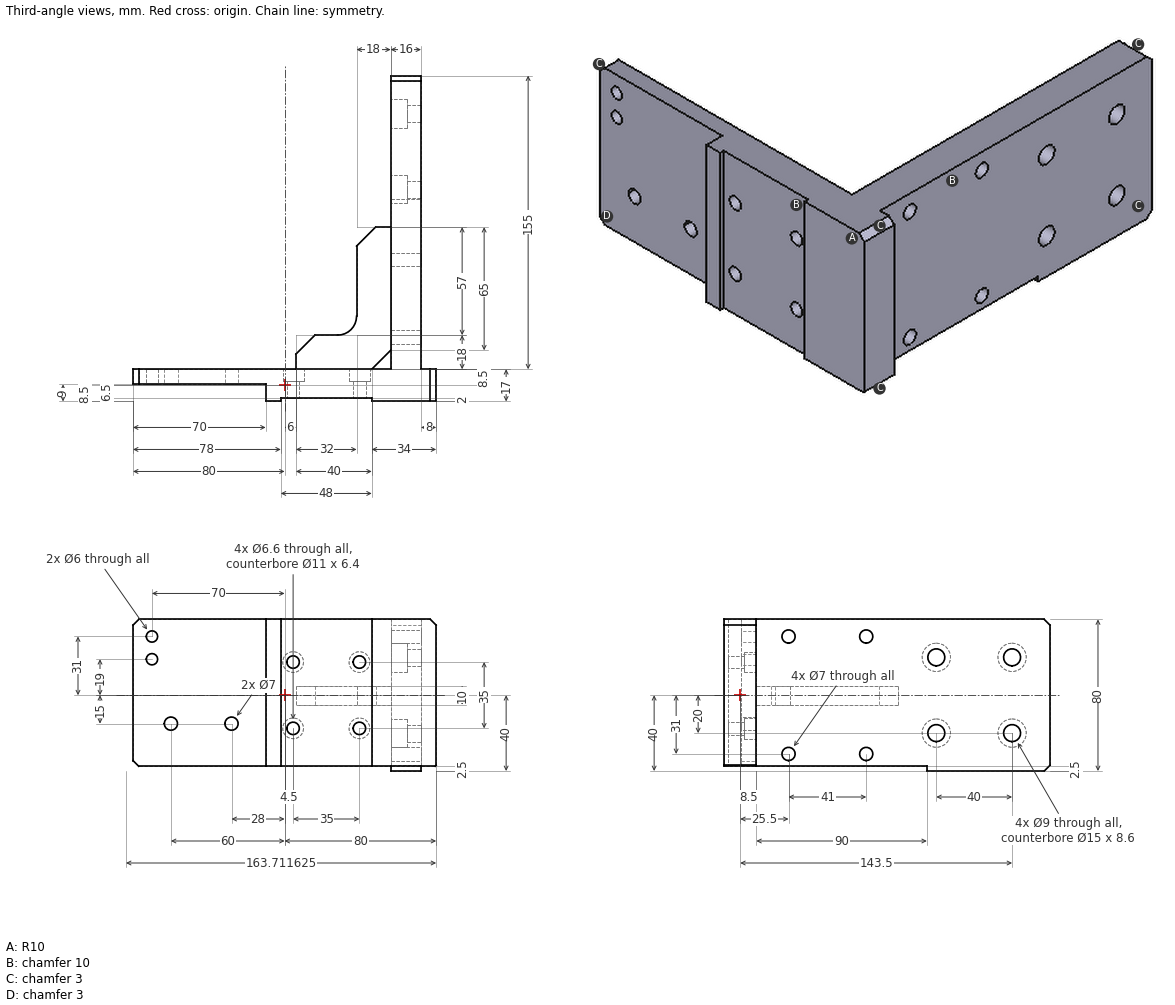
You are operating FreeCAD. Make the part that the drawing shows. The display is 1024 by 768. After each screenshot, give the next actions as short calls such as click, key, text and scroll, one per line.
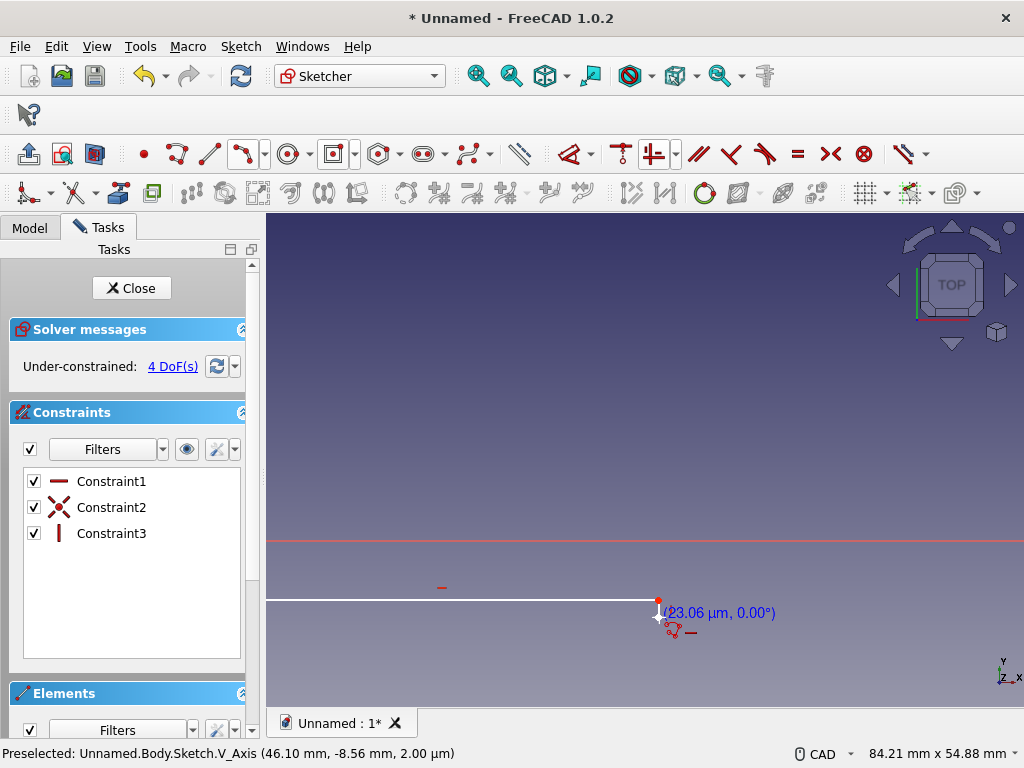
scroll(660, 616, down, 8)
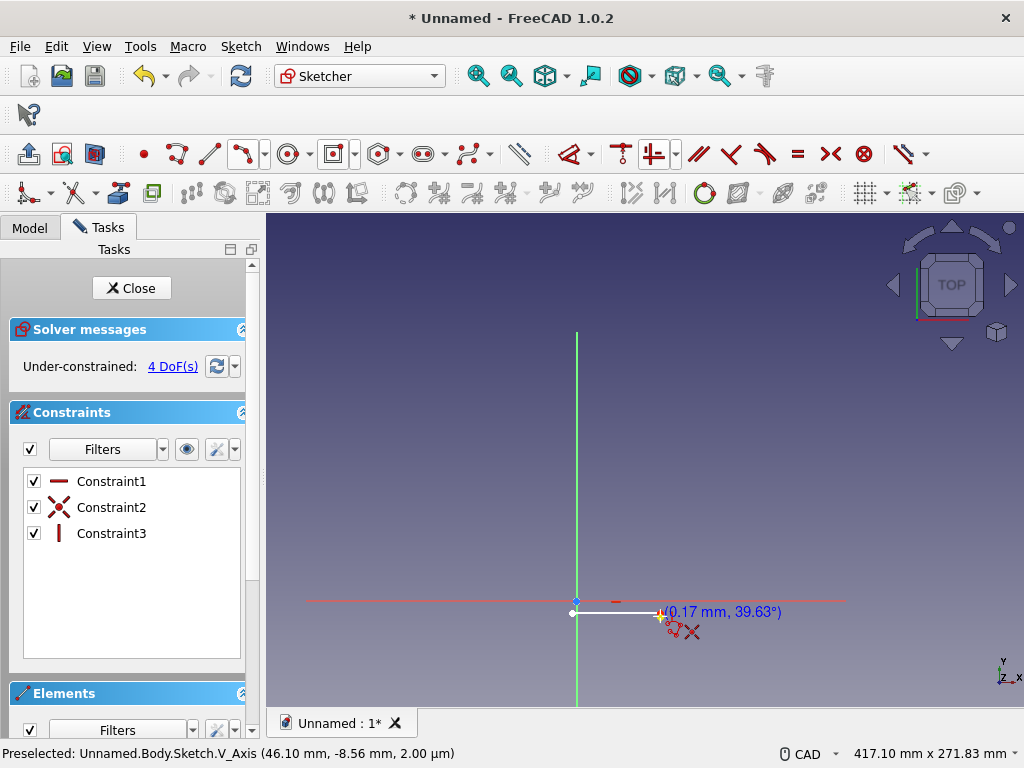
click(722, 617)
click(722, 586)
click(707, 586)
click(707, 304)
click(678, 304)
click(678, 586)
click(431, 586)
click(431, 617)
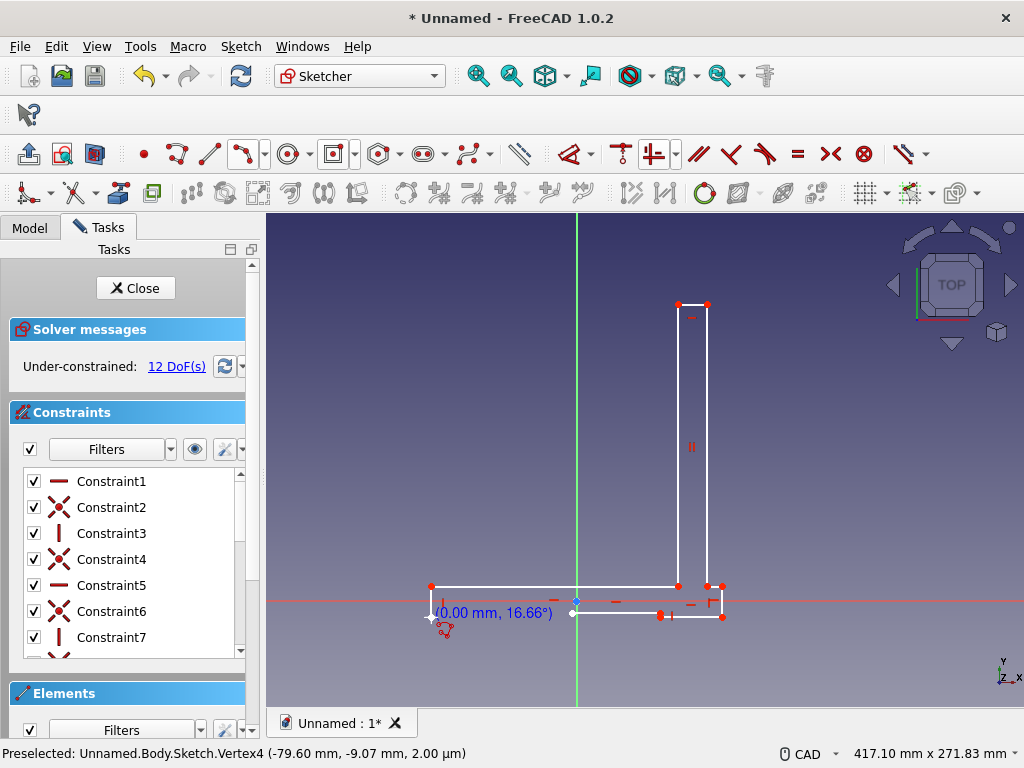
scroll(573, 617, up, 8)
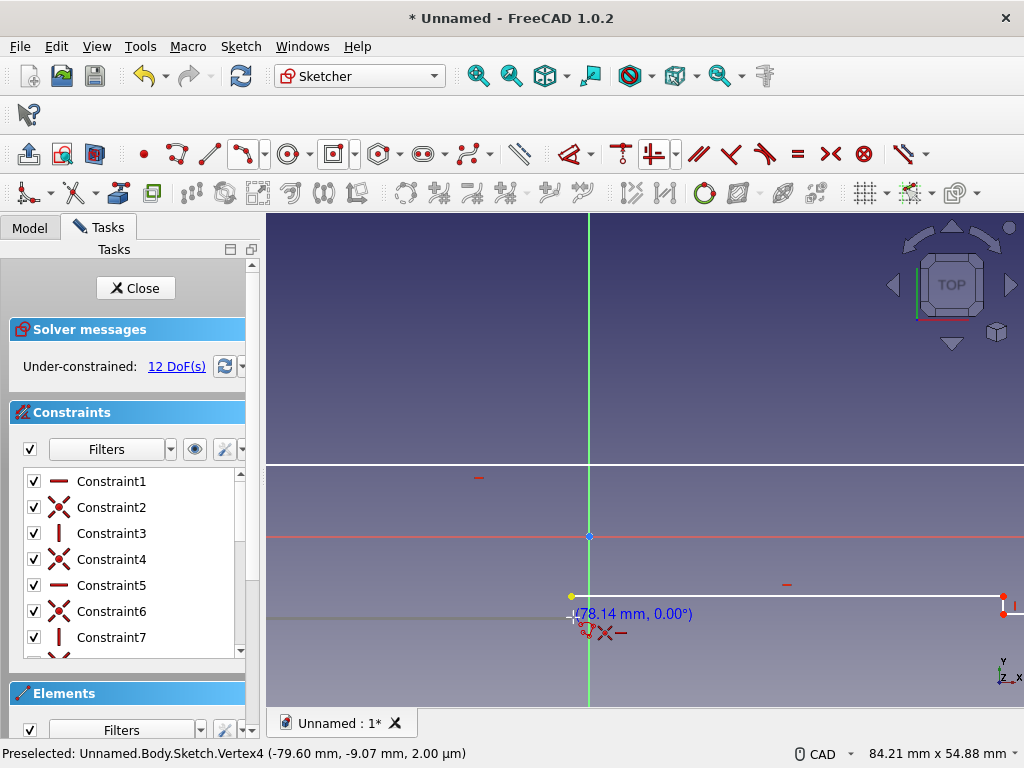
click(571, 614)
click(571, 596)
key(Escape)
key(Escape)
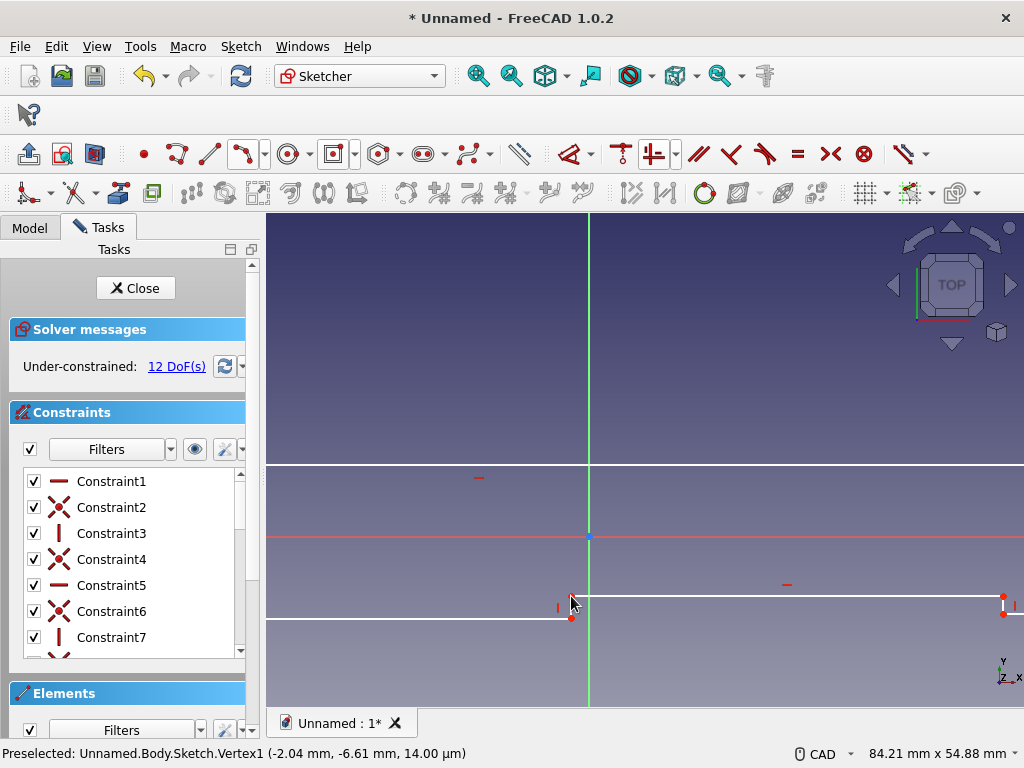
scroll(573, 617, down, 8)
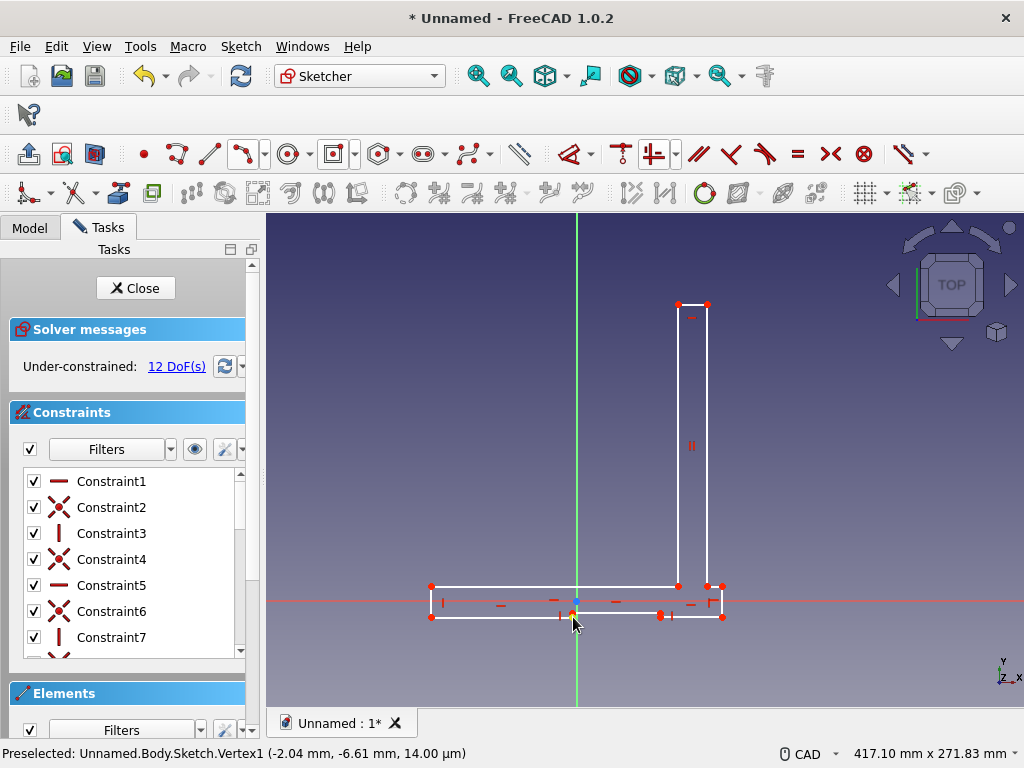
click(722, 587)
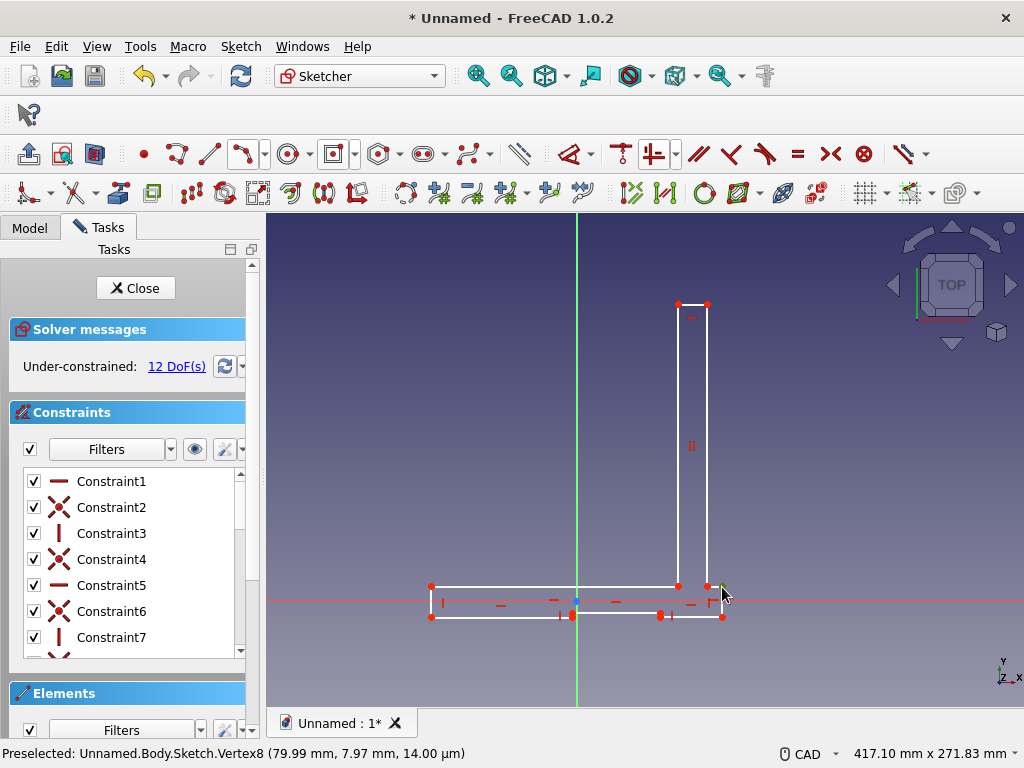
click(431, 587)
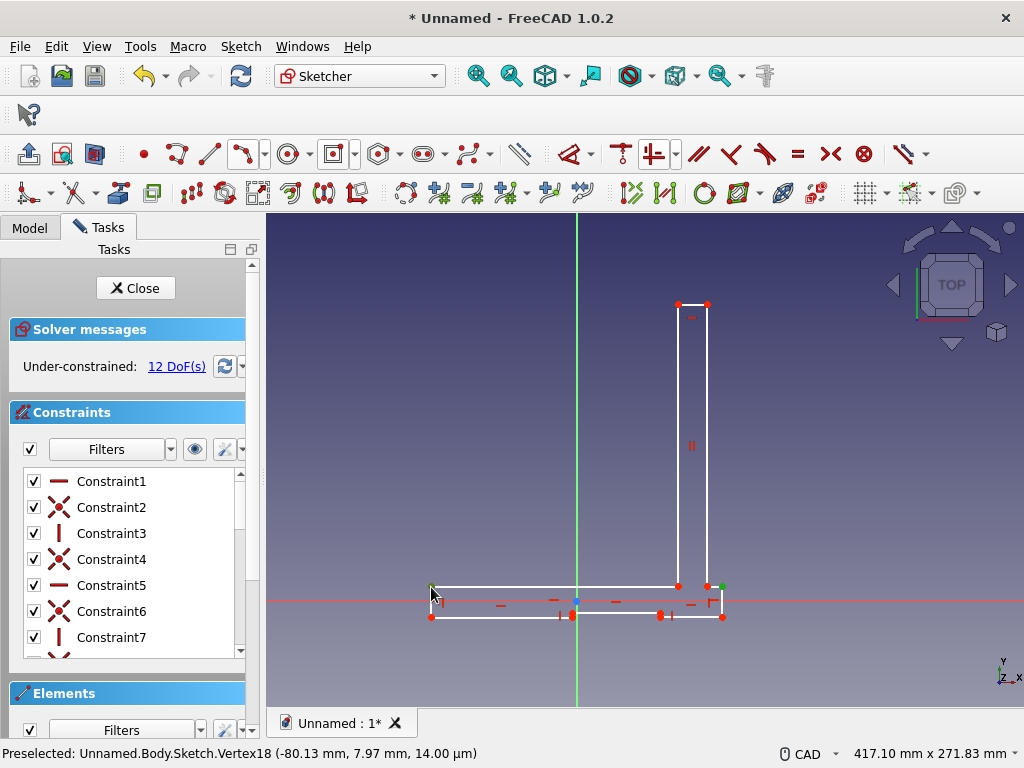
click(577, 554)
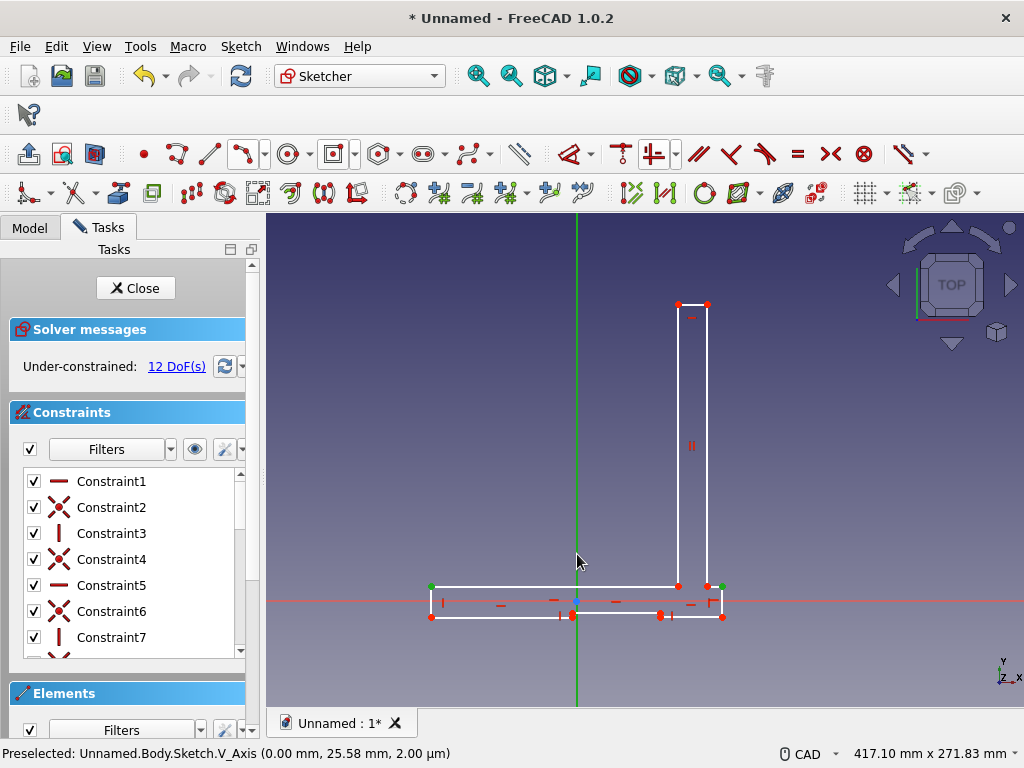
click(831, 154)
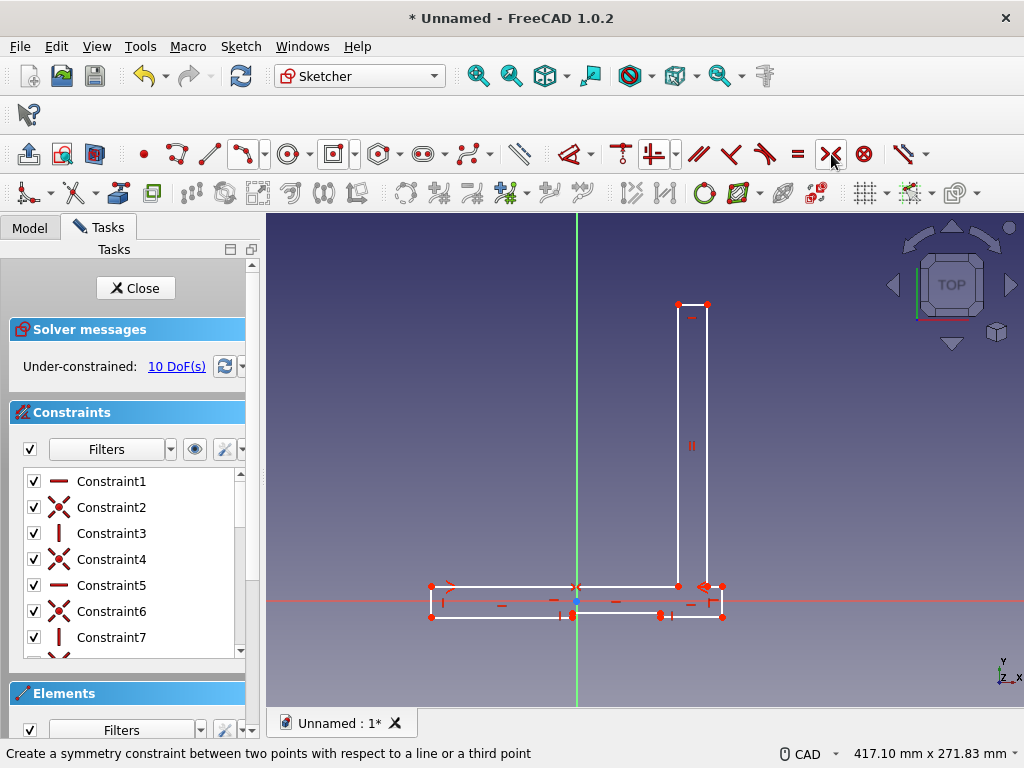
scroll(660, 615, up, 12)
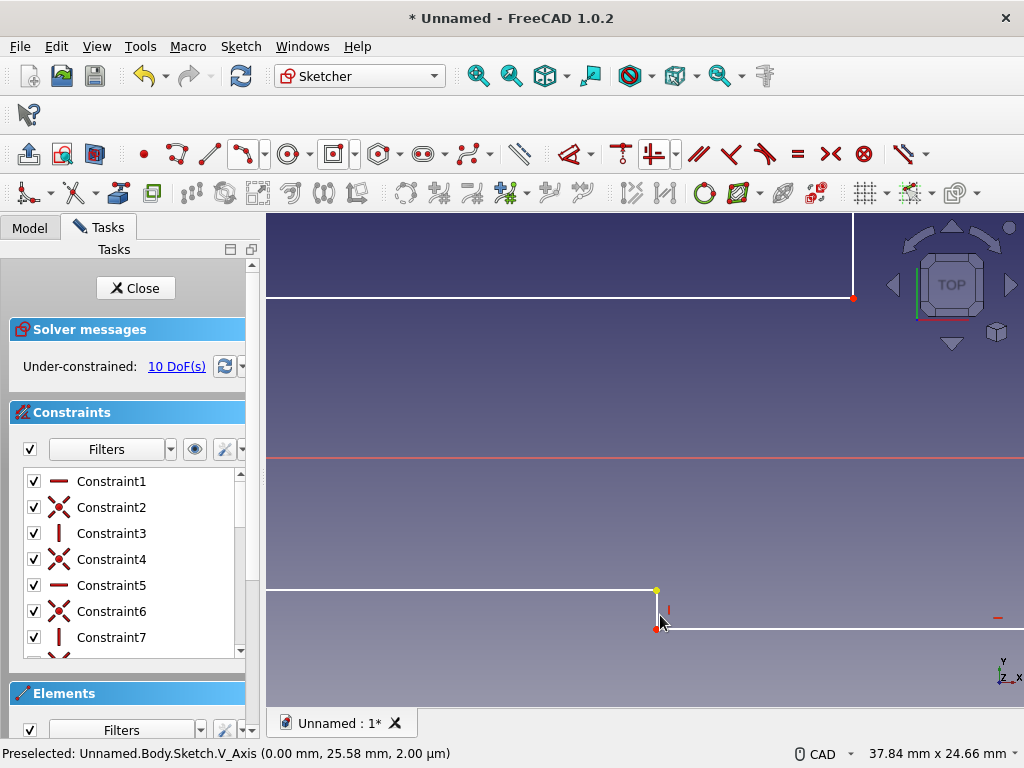
click(657, 610)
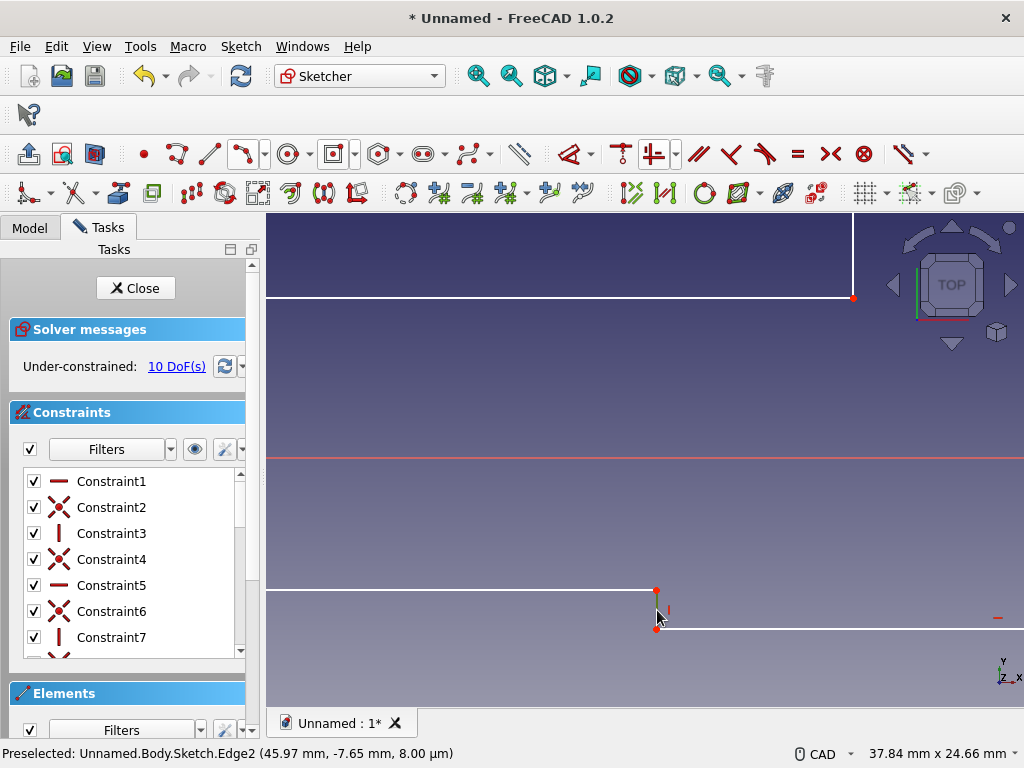
key(i)